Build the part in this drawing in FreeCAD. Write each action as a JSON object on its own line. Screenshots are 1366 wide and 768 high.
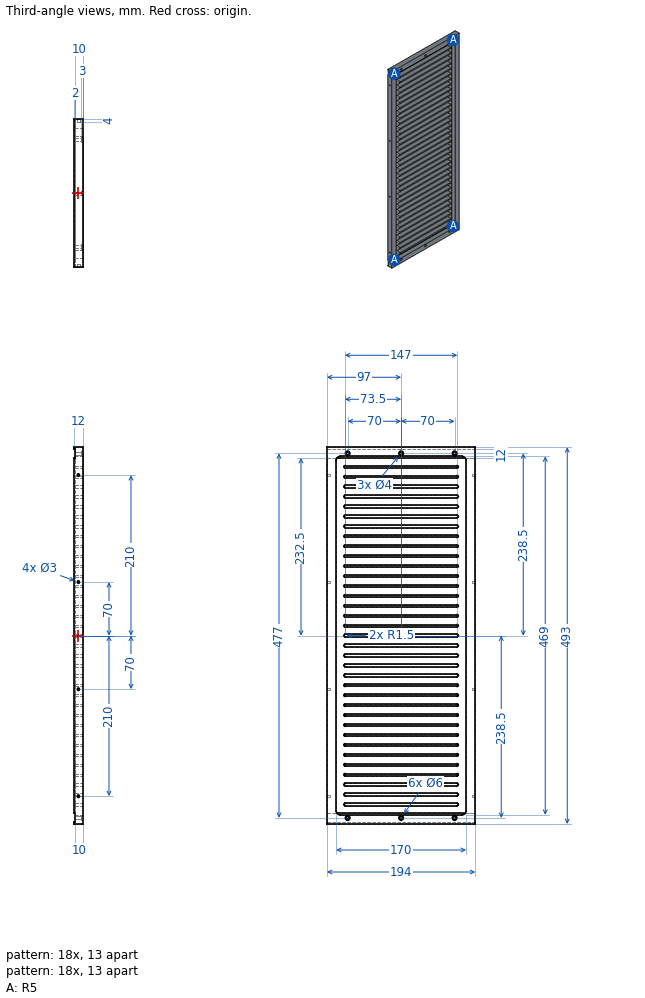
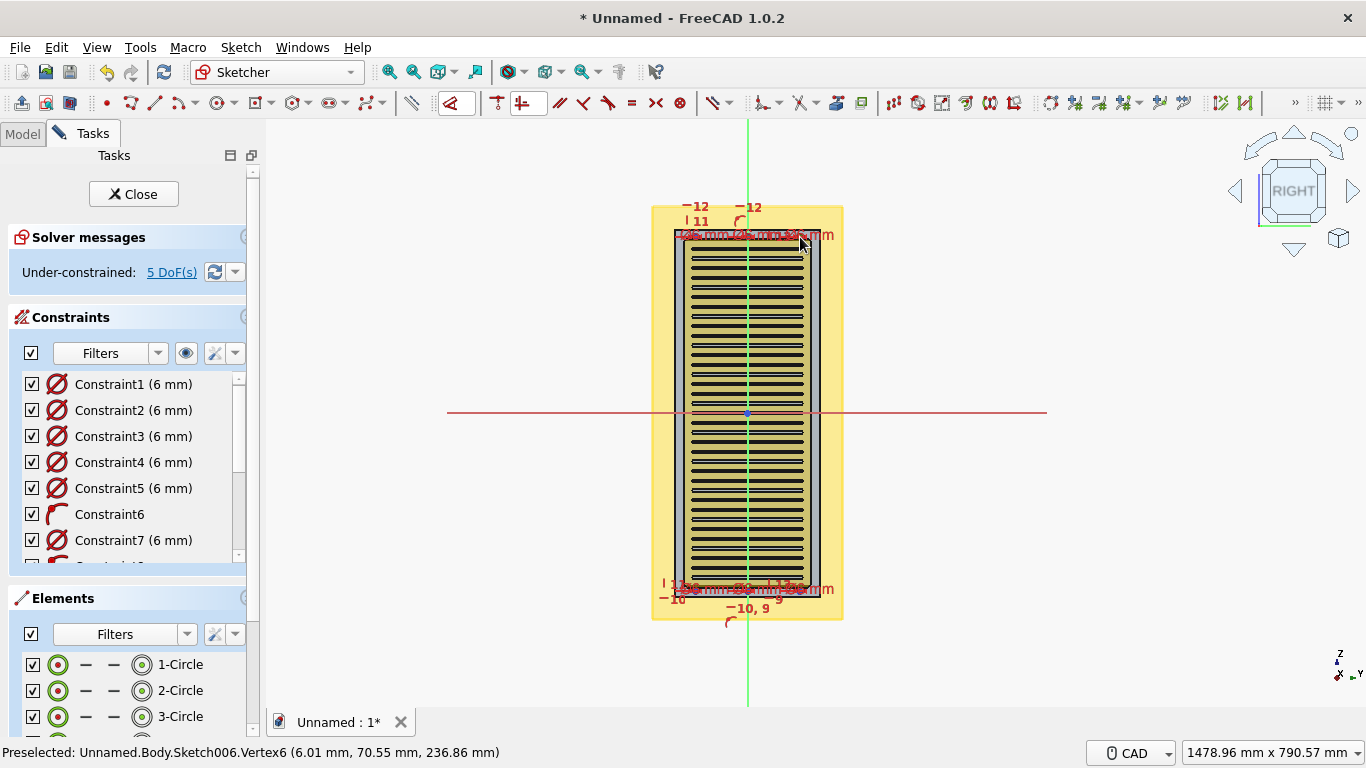
{"action": "left_click", "coordinate": [542, 104]}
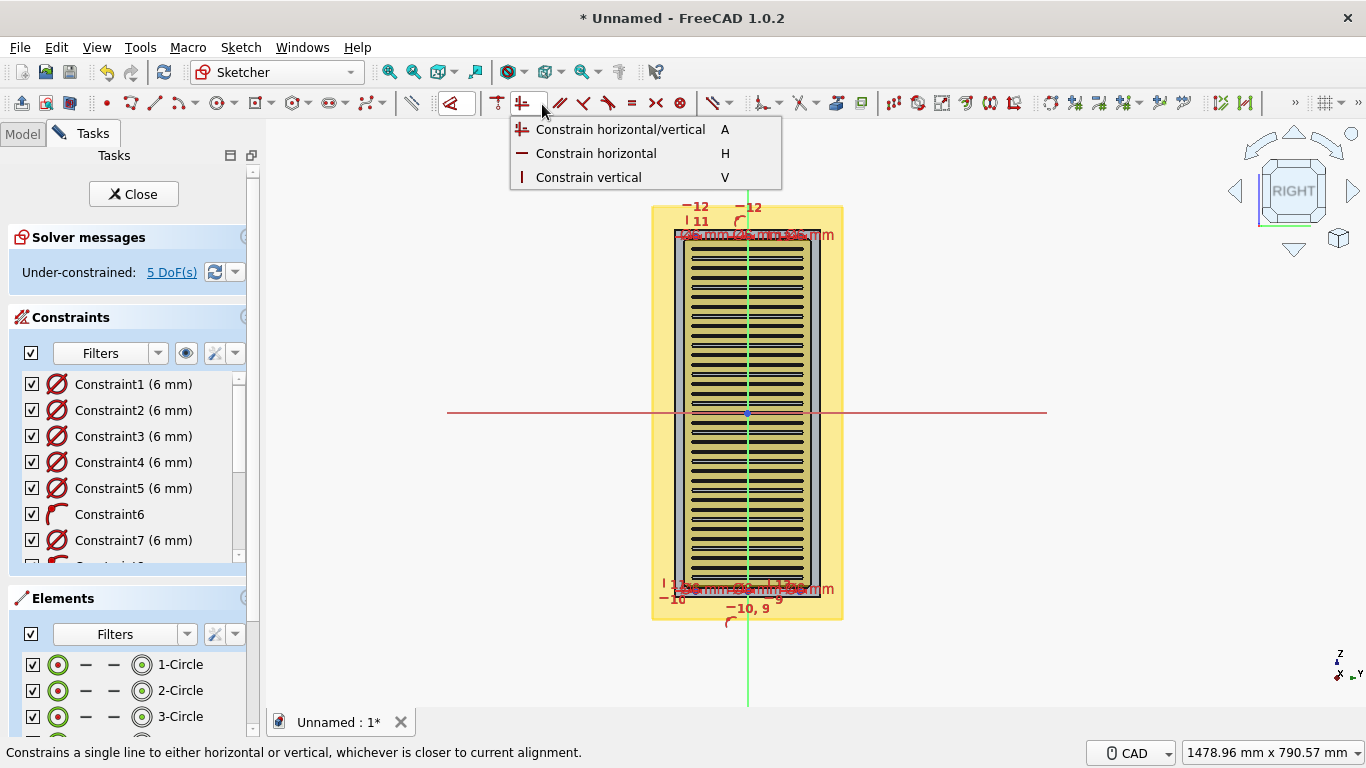
{"action": "left_click", "coordinate": [646, 153]}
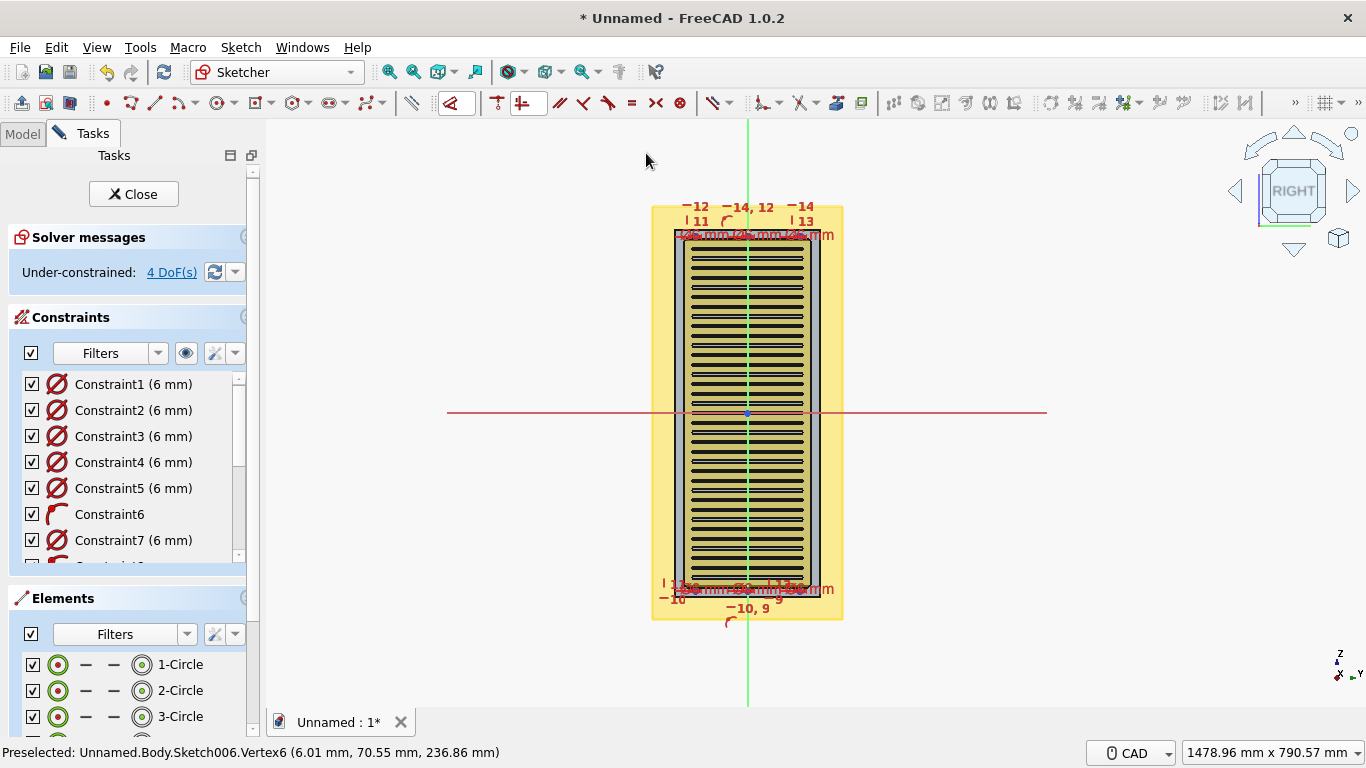
{"action": "left_click", "coordinate": [800, 591]}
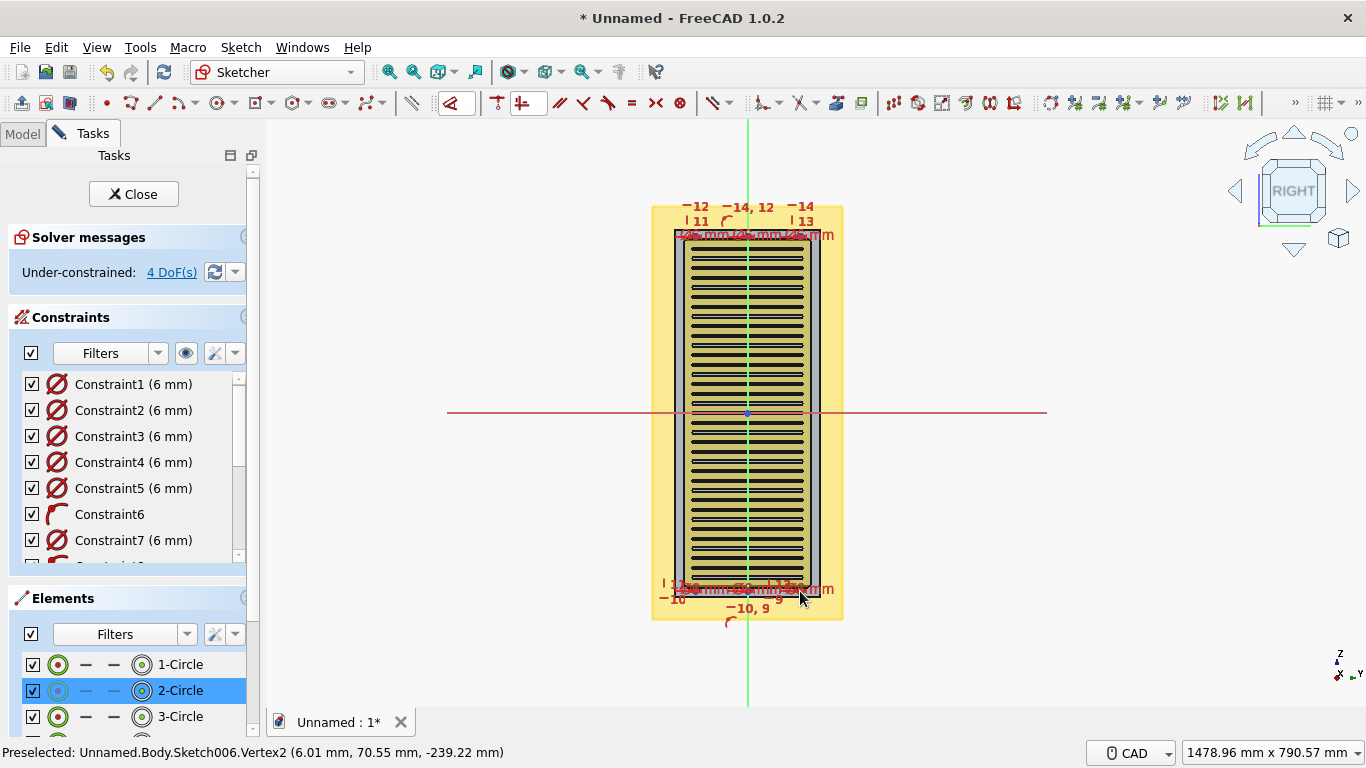
{"action": "key", "text": "l"}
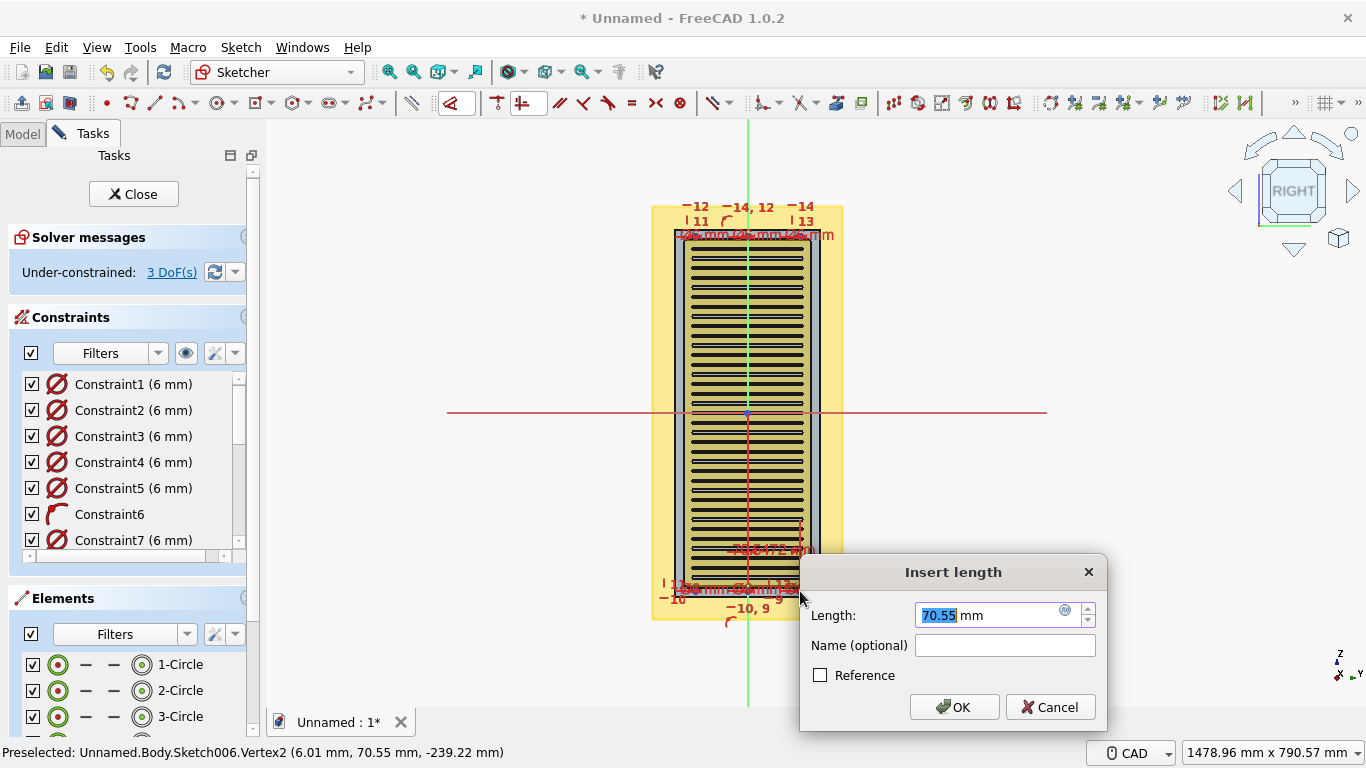
{"action": "type", "text": "70"}
{"action": "key", "text": "Return"}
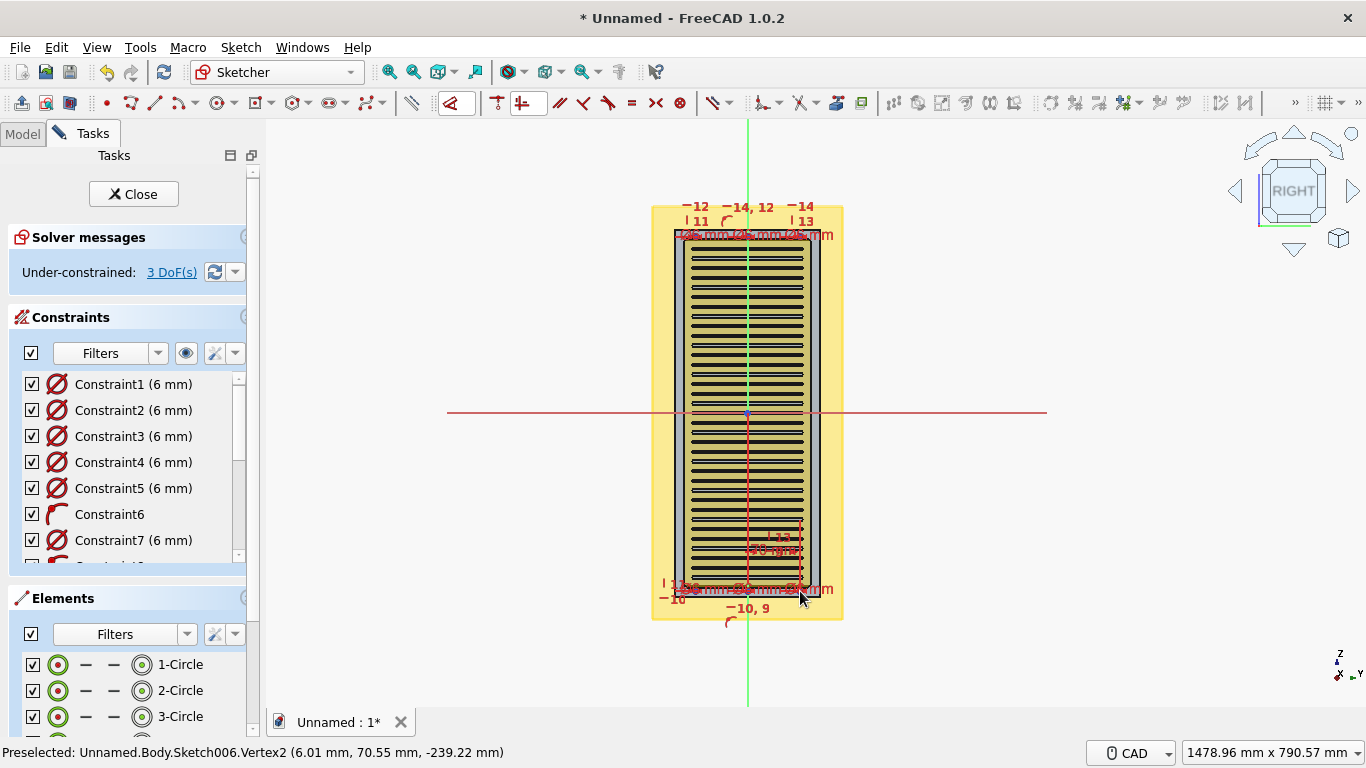
{"action": "left_click", "coordinate": [695, 591]}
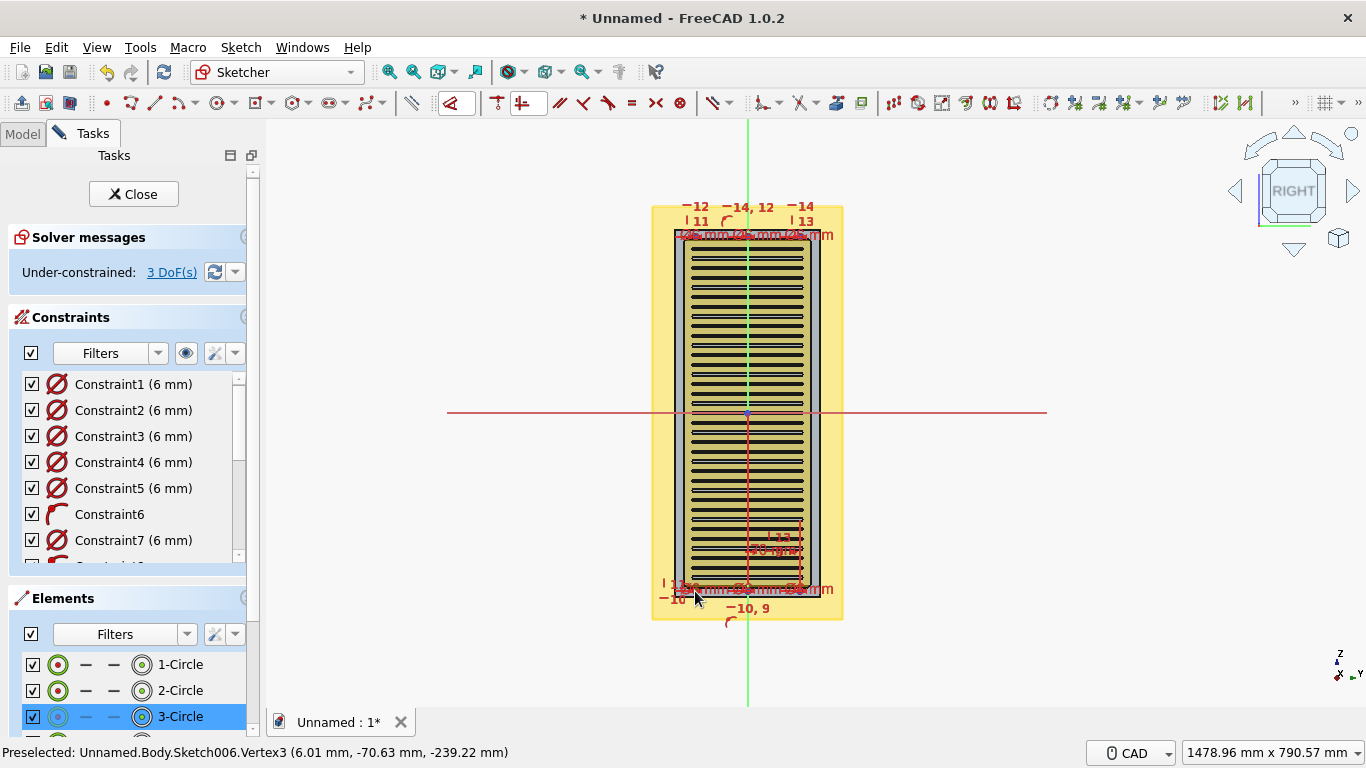
{"action": "left_click", "coordinate": [470, 104]}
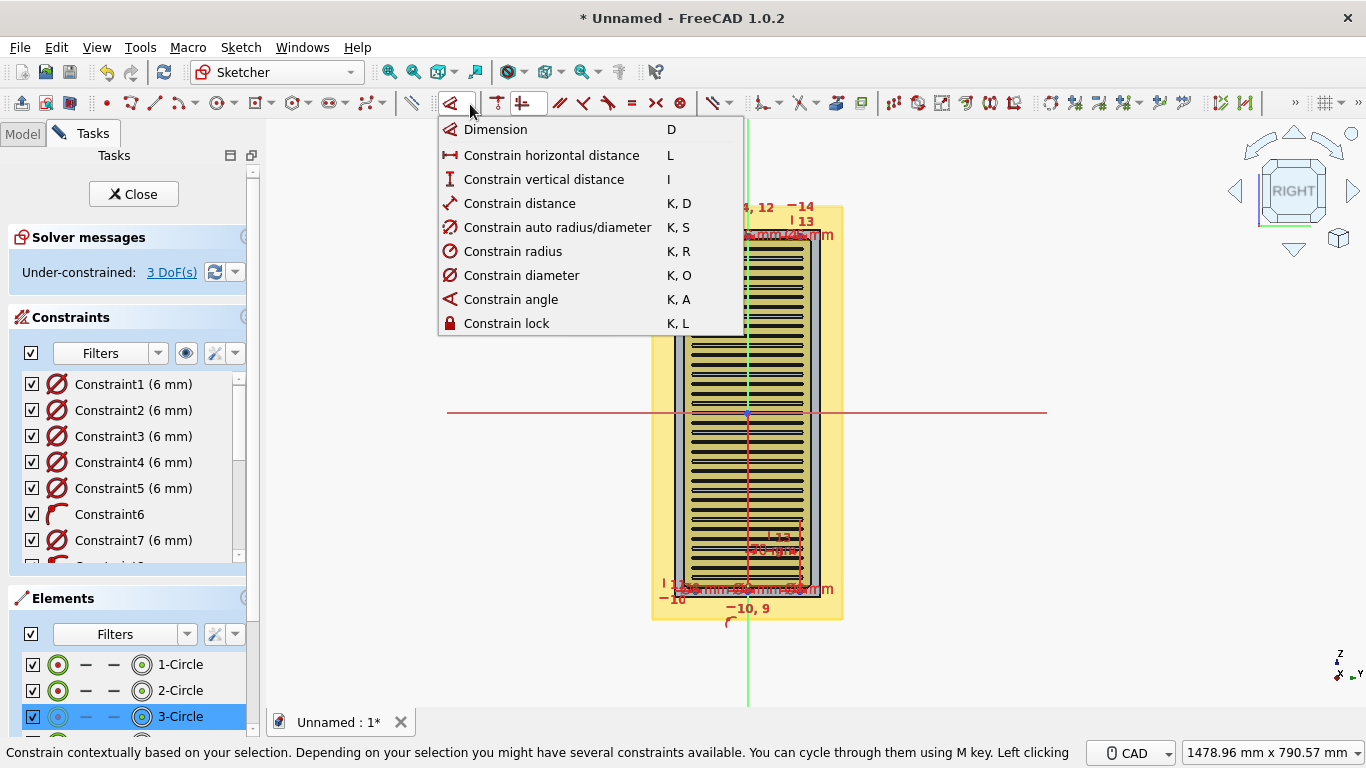
{"action": "left_click", "coordinate": [591, 155]}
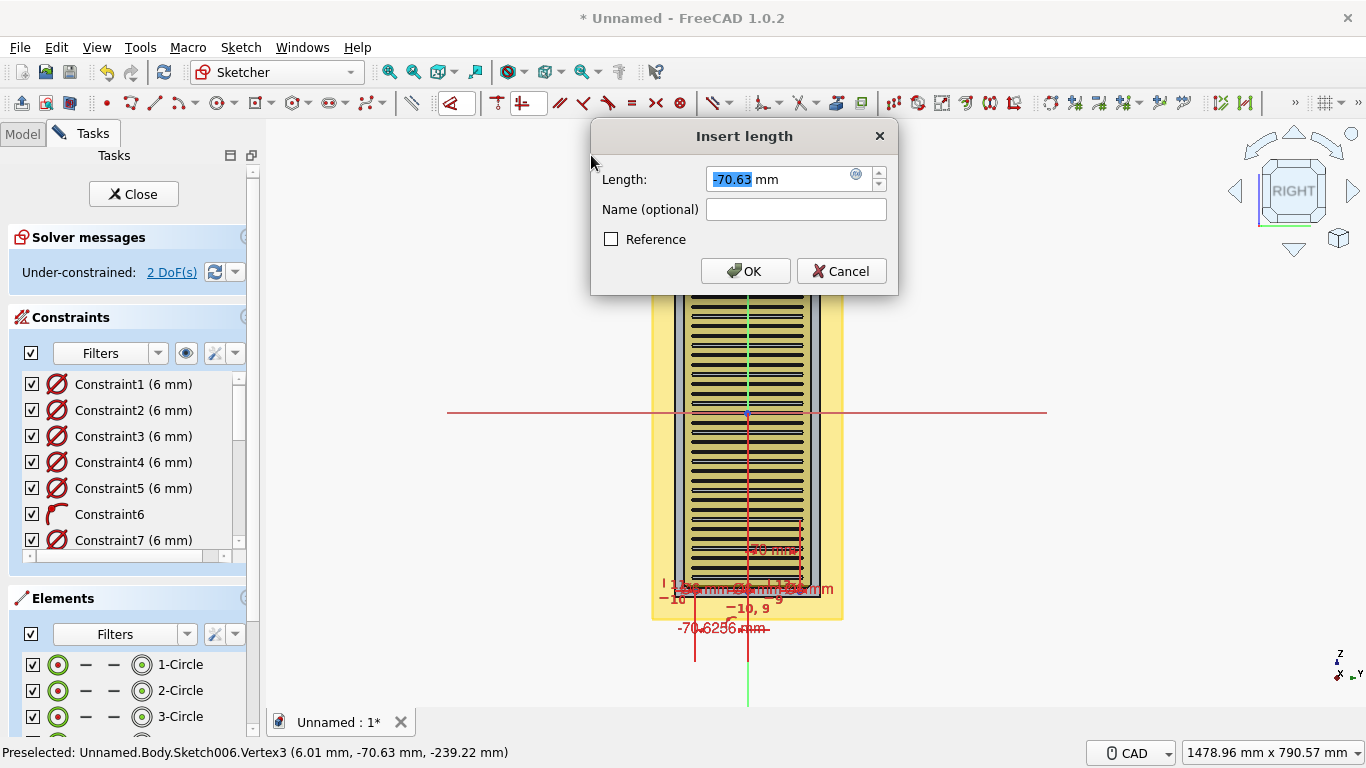
{"action": "type", "text": "-70"}
{"action": "key", "text": "Return"}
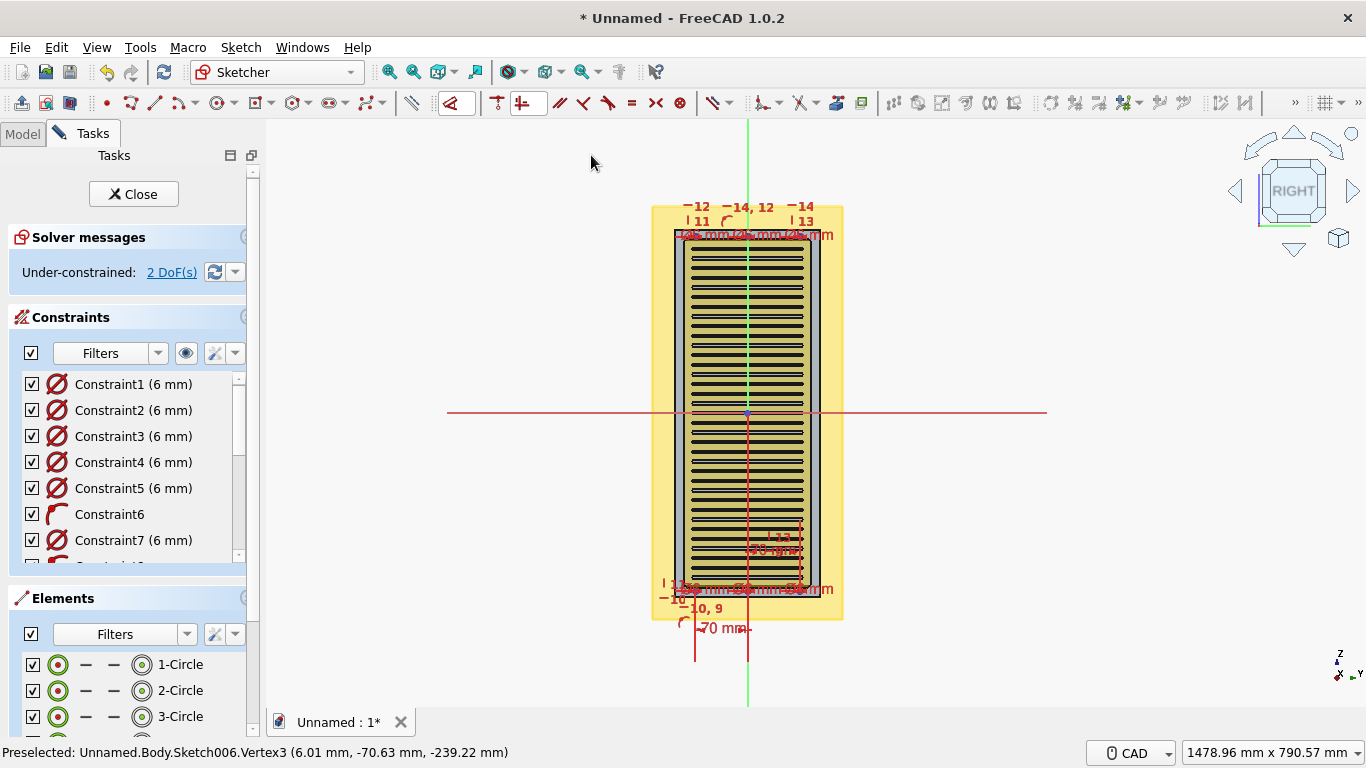
{"action": "left_click", "coordinate": [695, 591]}